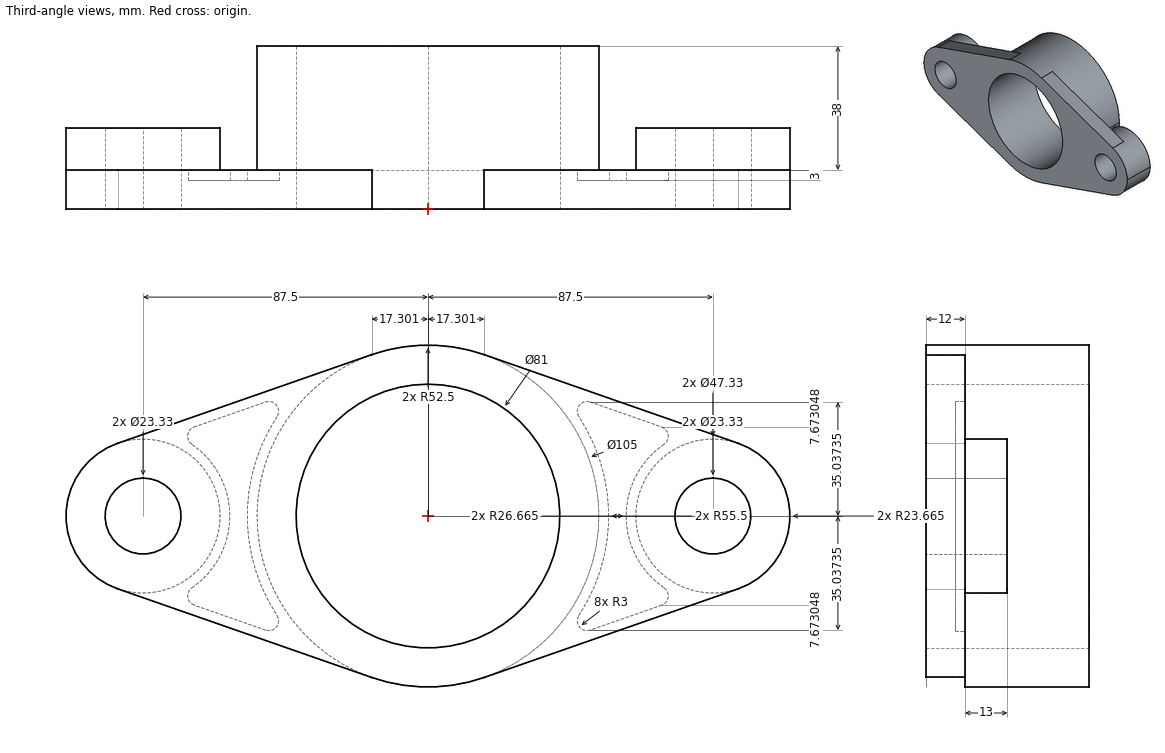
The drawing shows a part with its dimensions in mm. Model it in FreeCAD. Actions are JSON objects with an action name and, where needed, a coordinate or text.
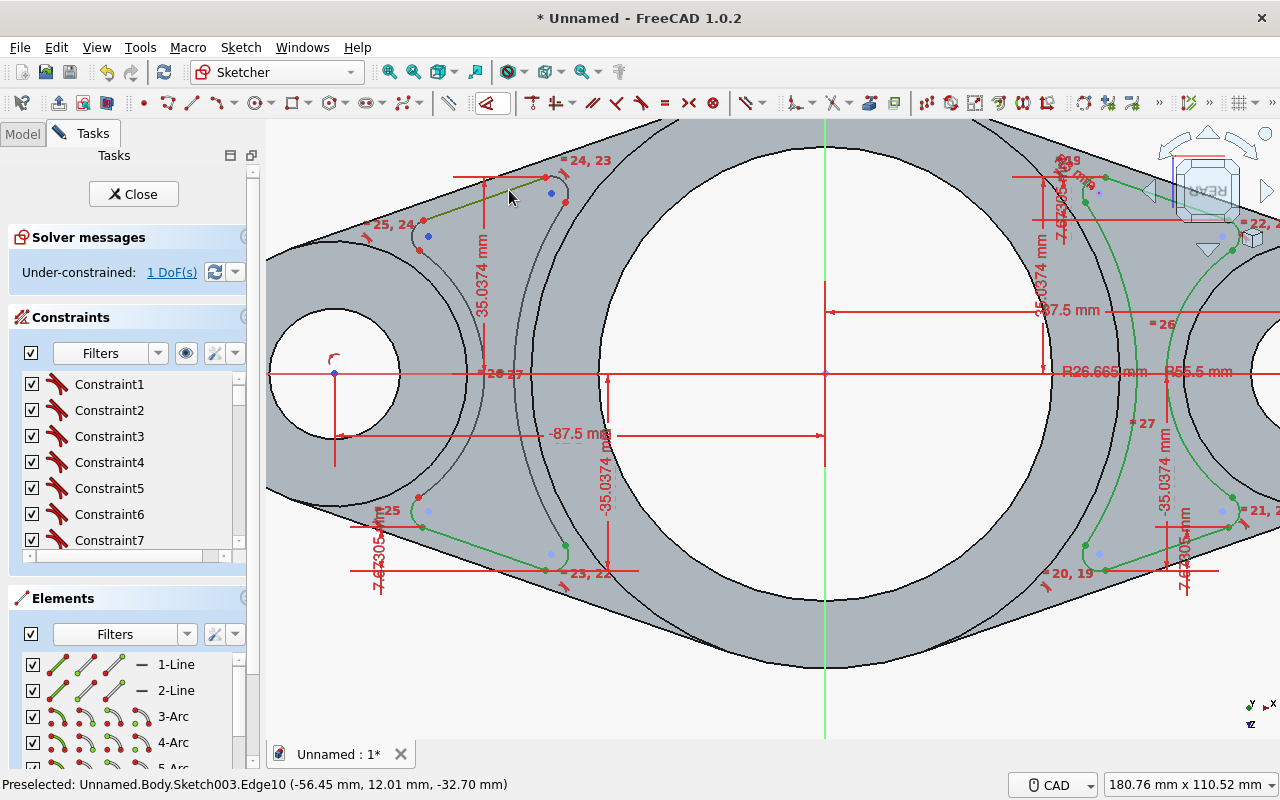
{"action": "key", "text": "i"}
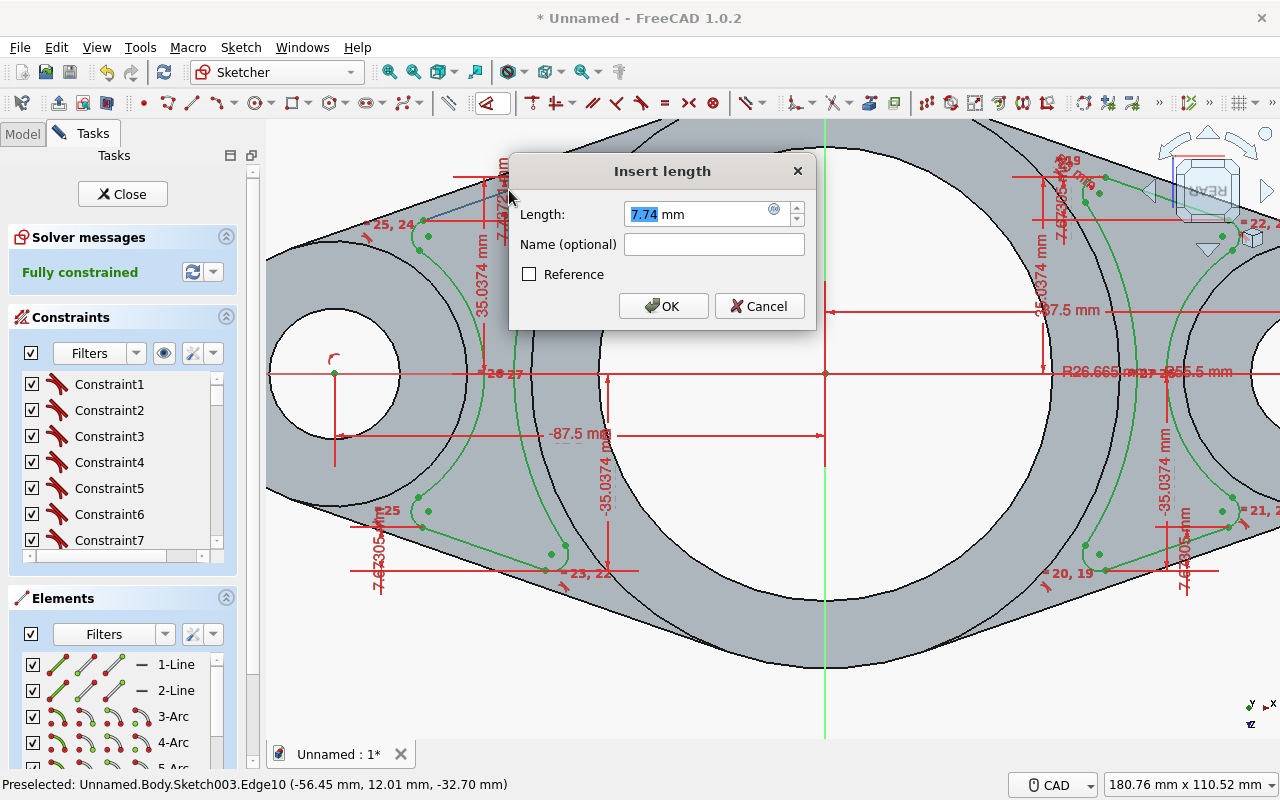
{"action": "type", "text": "7.673048"}
{"action": "key", "text": "Return"}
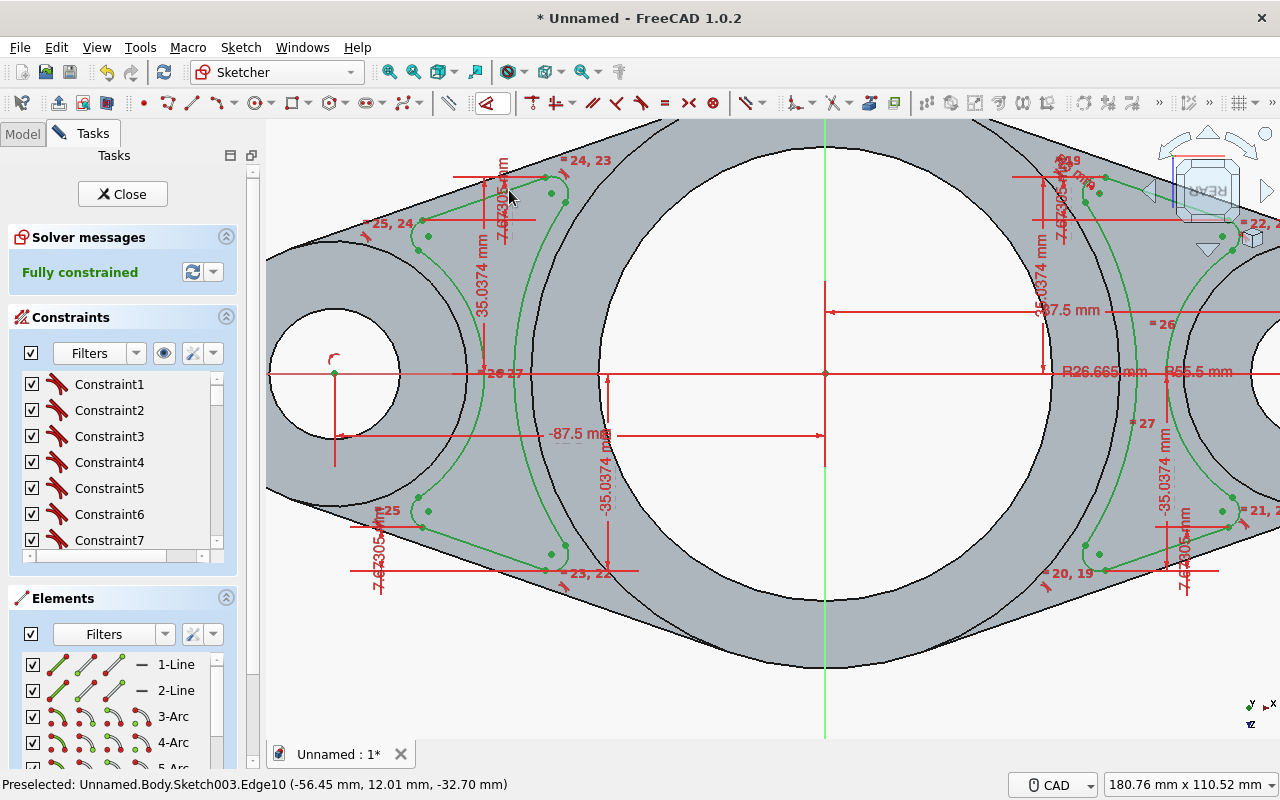
{"action": "left_click", "coordinate": [123, 194]}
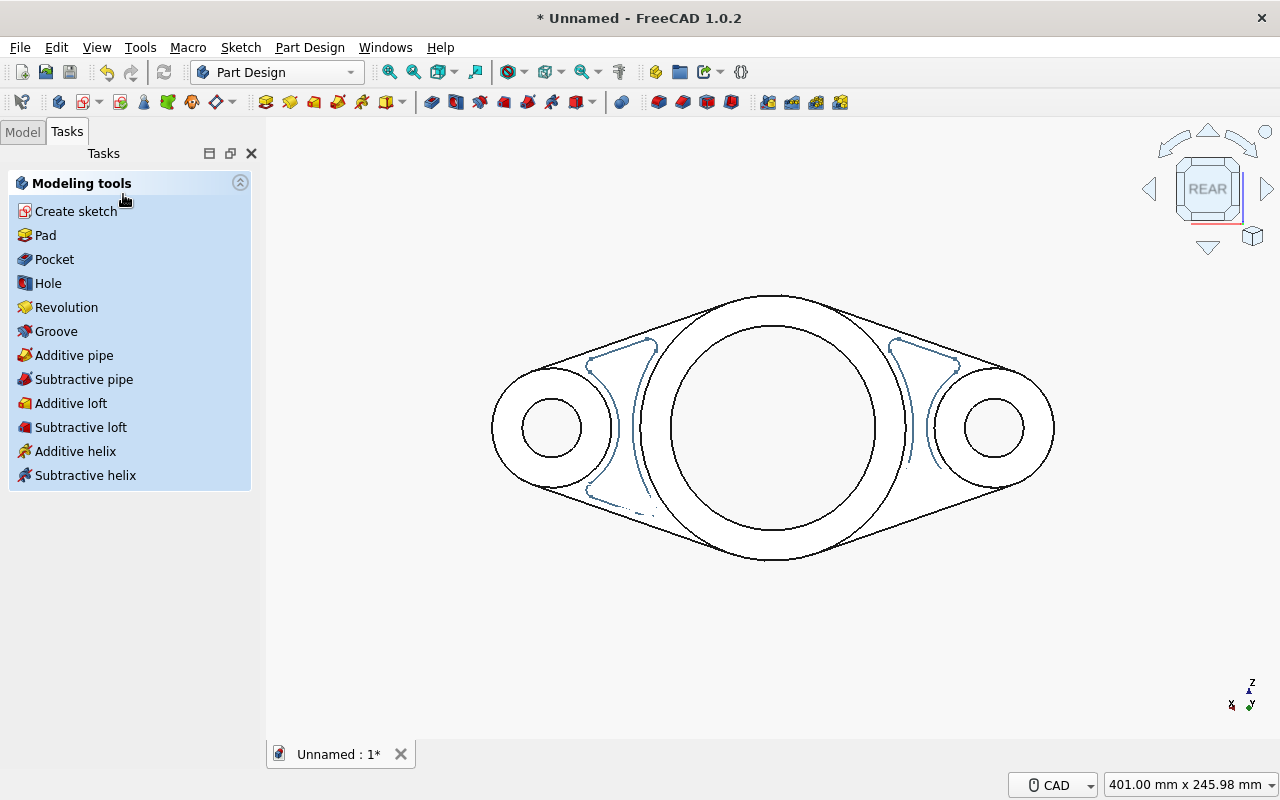
{"action": "left_click", "coordinate": [432, 102]}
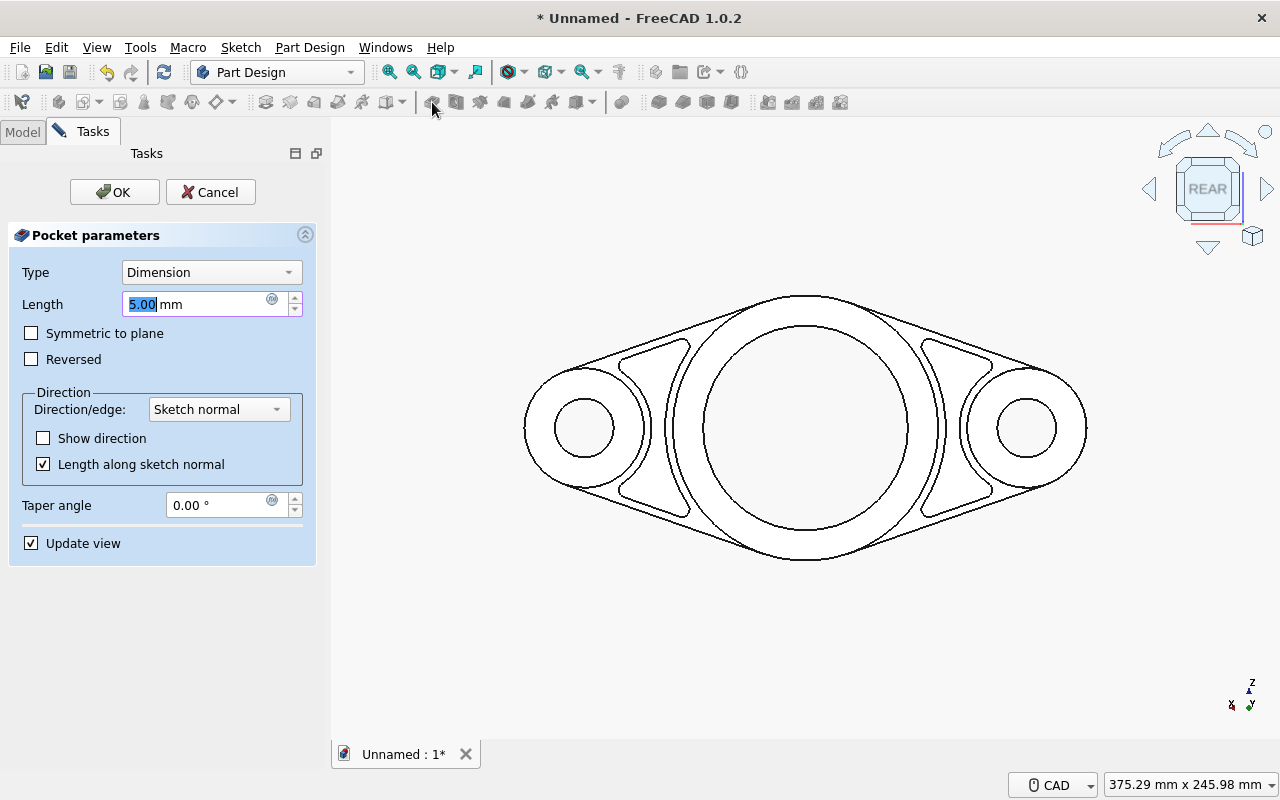
{"action": "type", "text": "3"}
{"action": "key", "text": "Tab"}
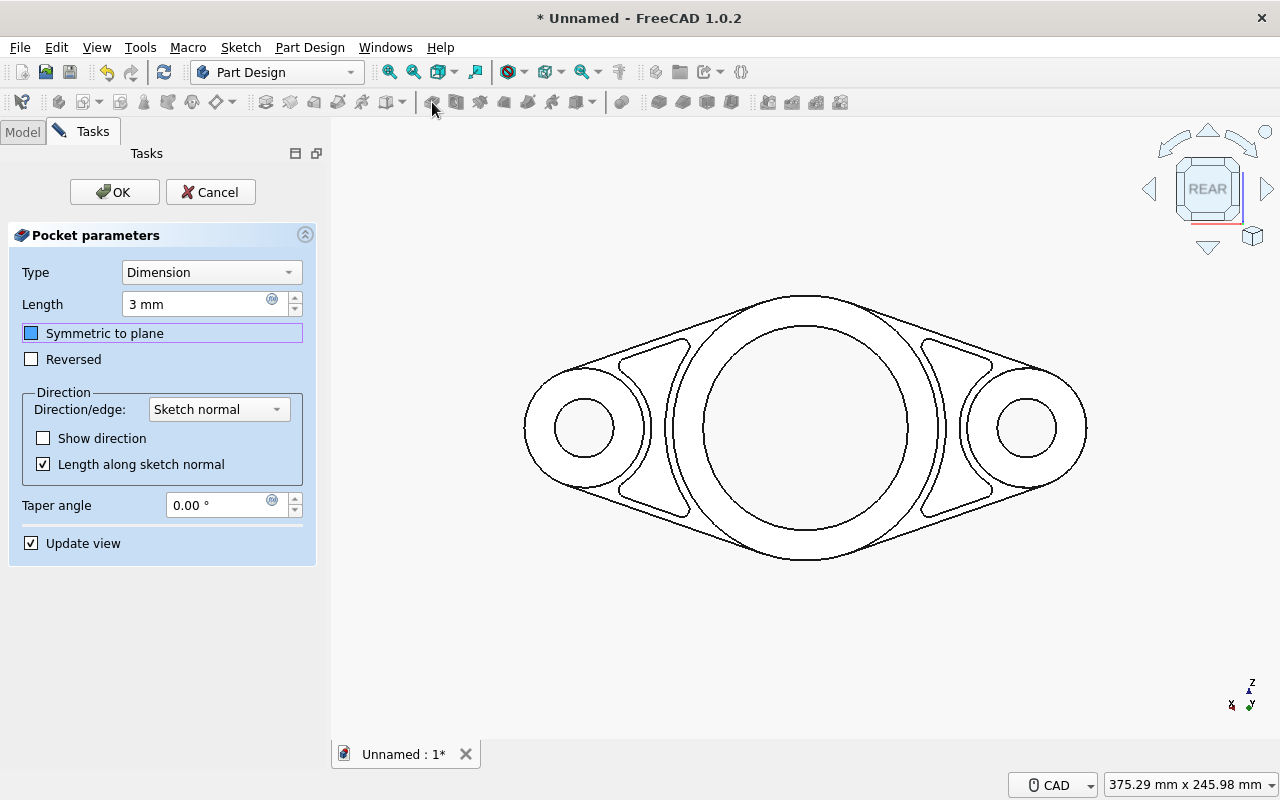
{"action": "left_click", "coordinate": [115, 192]}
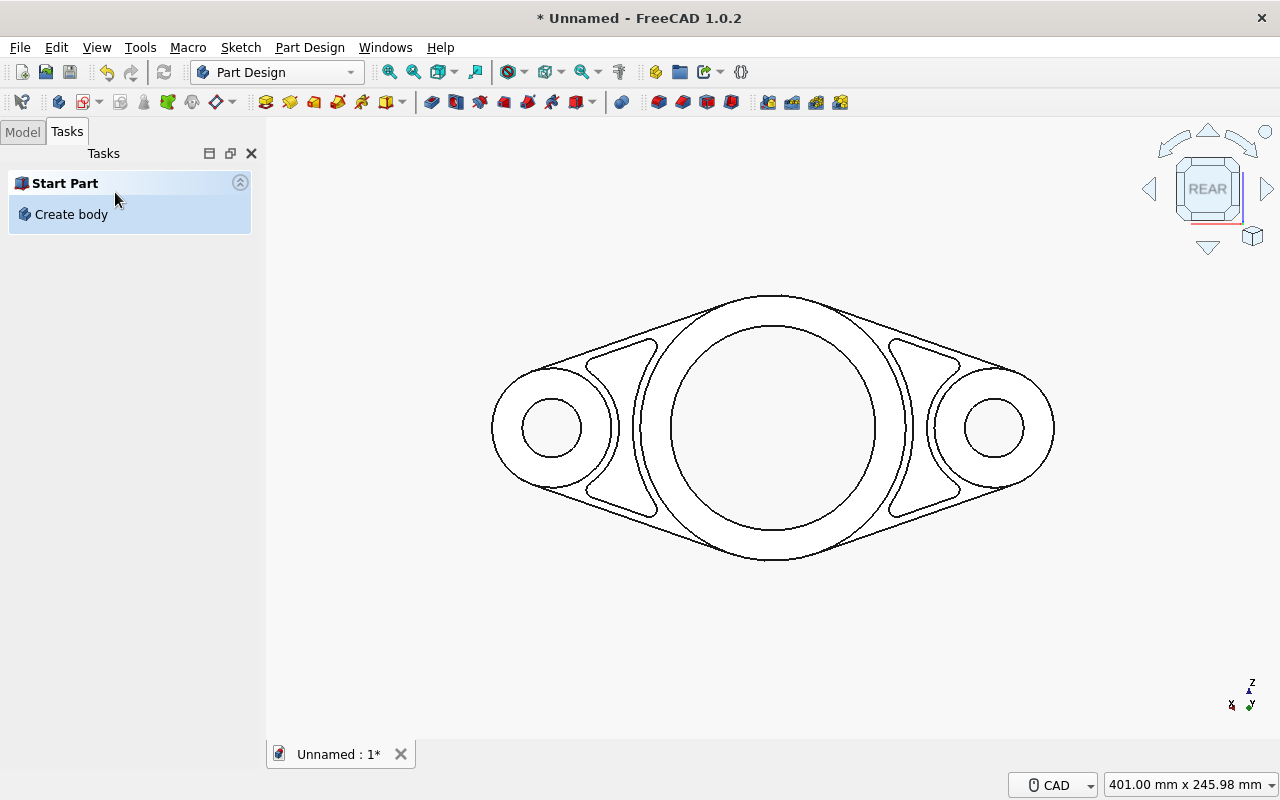
{"action": "key", "text": "0"}